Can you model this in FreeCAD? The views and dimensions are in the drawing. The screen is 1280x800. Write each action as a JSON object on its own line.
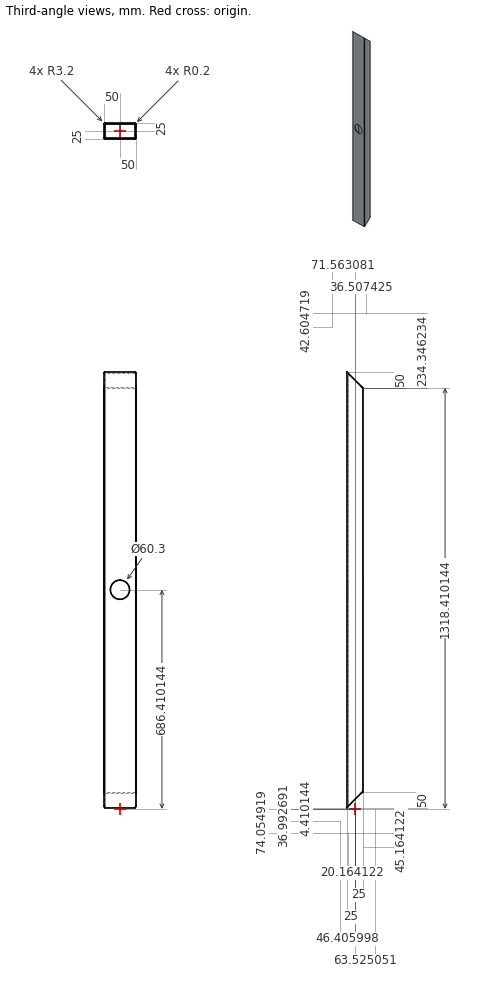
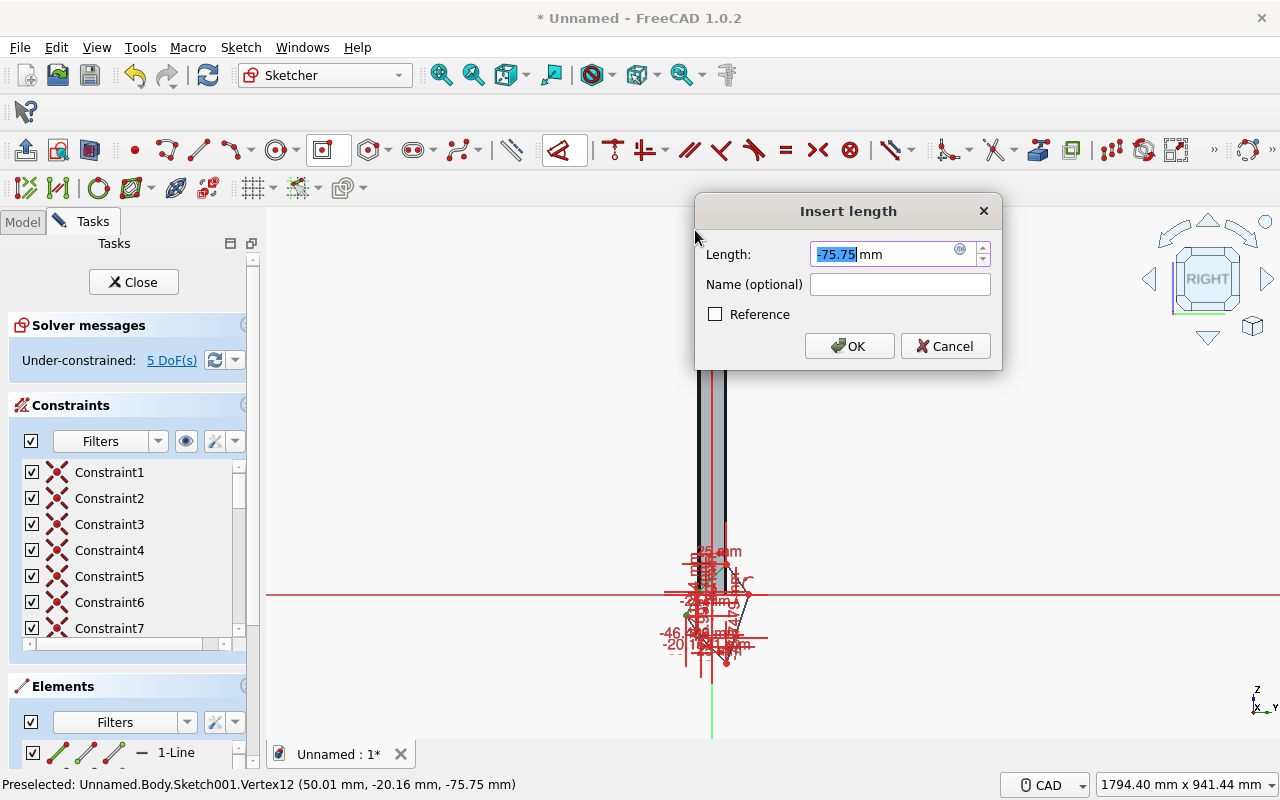
{"action": "type", "text": "-74.054919"}
{"action": "key", "text": "Return"}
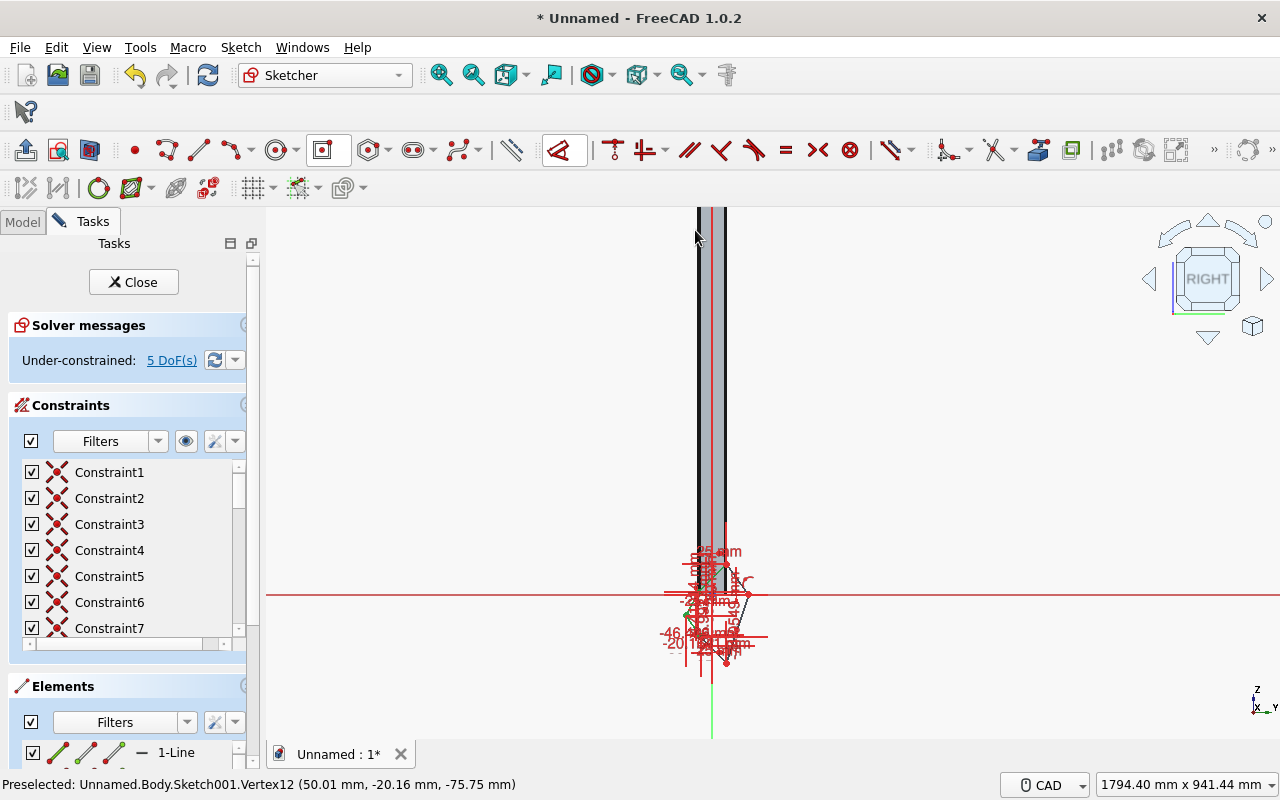
{"action": "left_click", "coordinate": [749, 595]}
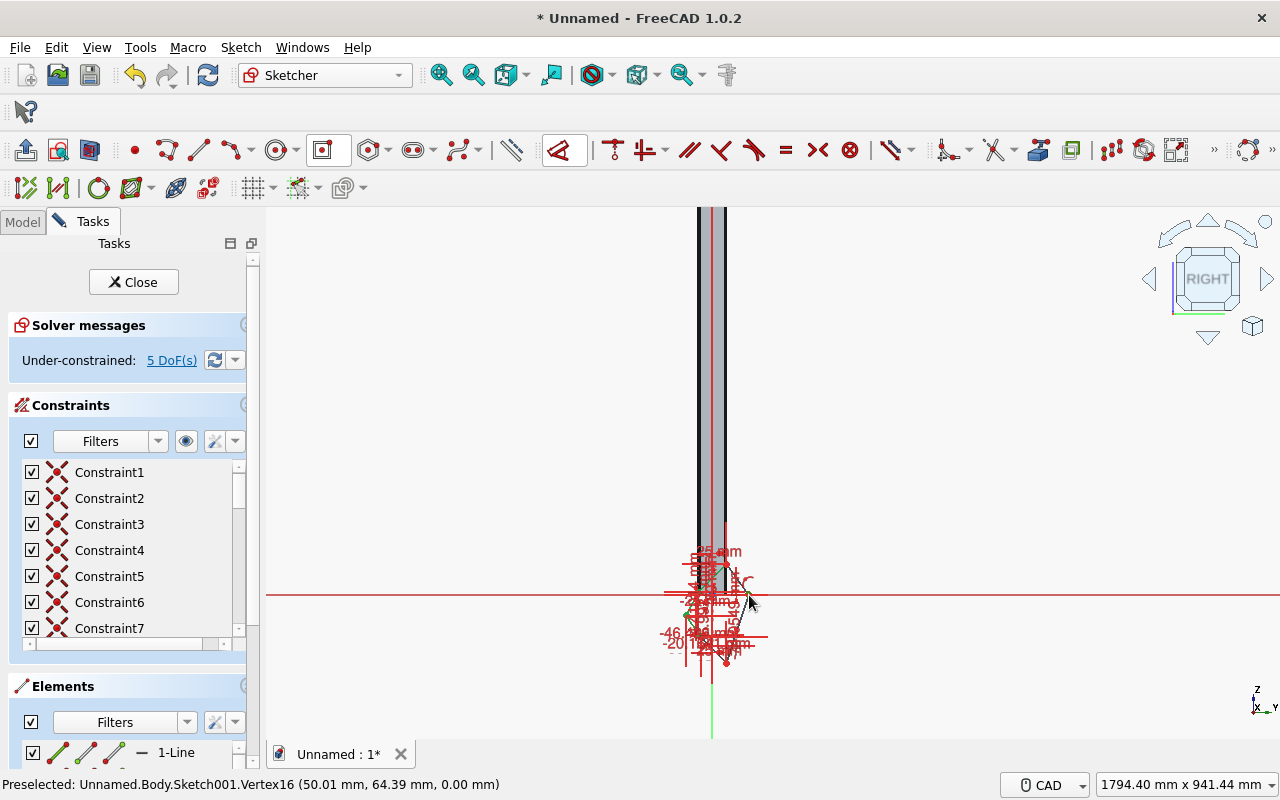
{"action": "left_click", "coordinate": [582, 150]}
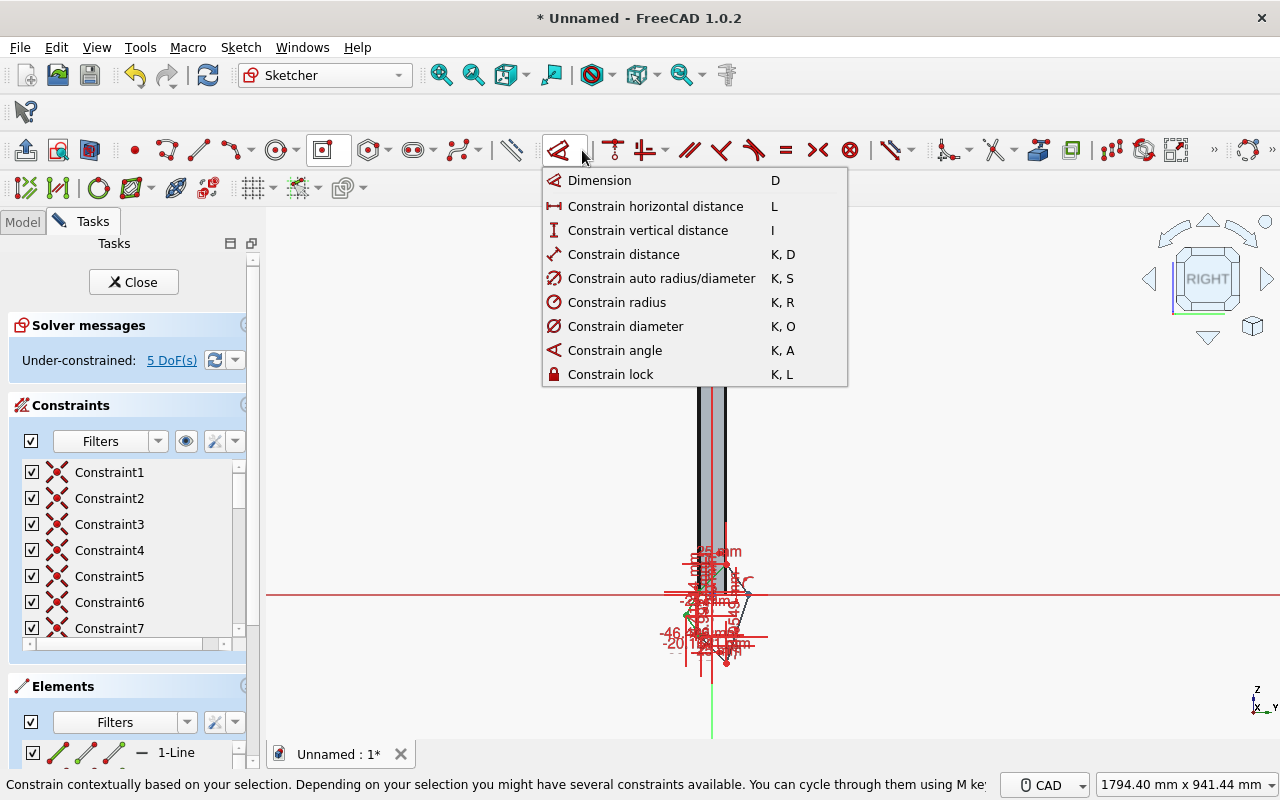
{"action": "left_click", "coordinate": [695, 206]}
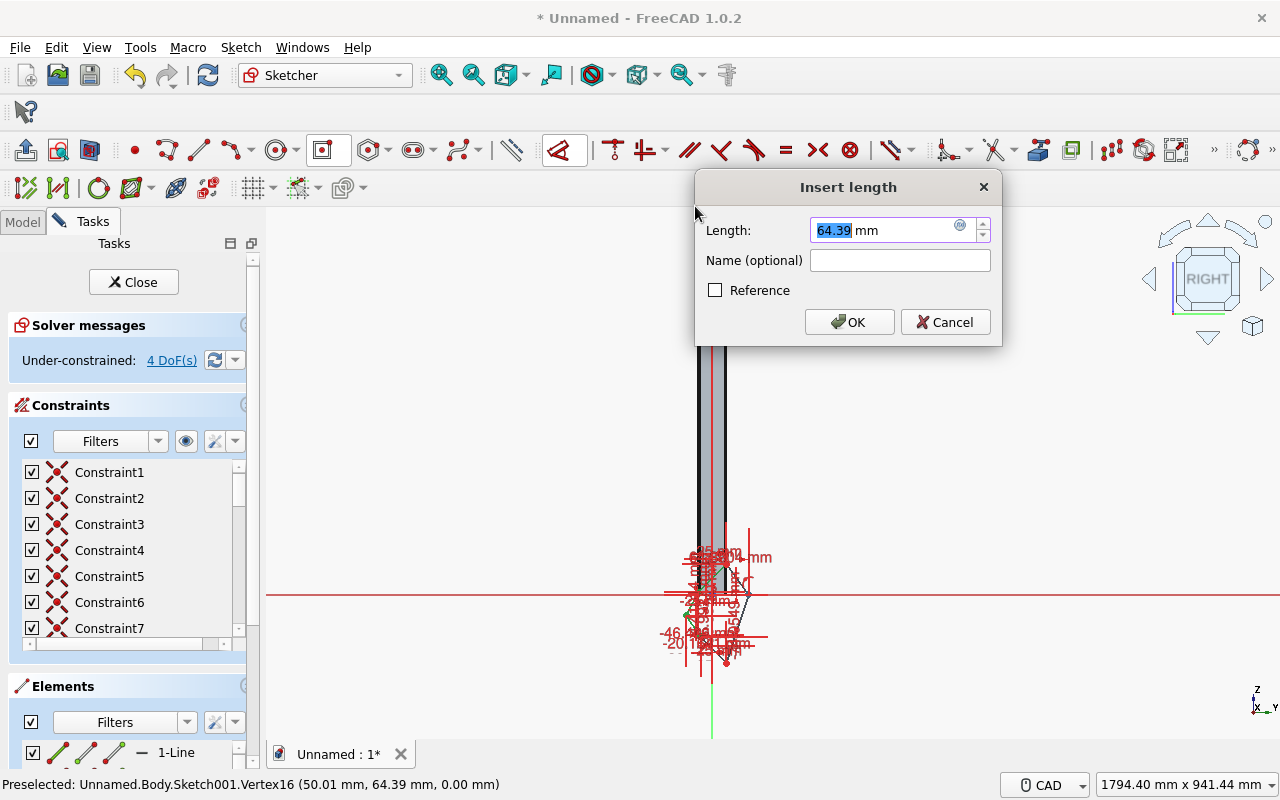
{"action": "type", "text": "63.525051"}
{"action": "key", "text": "Return"}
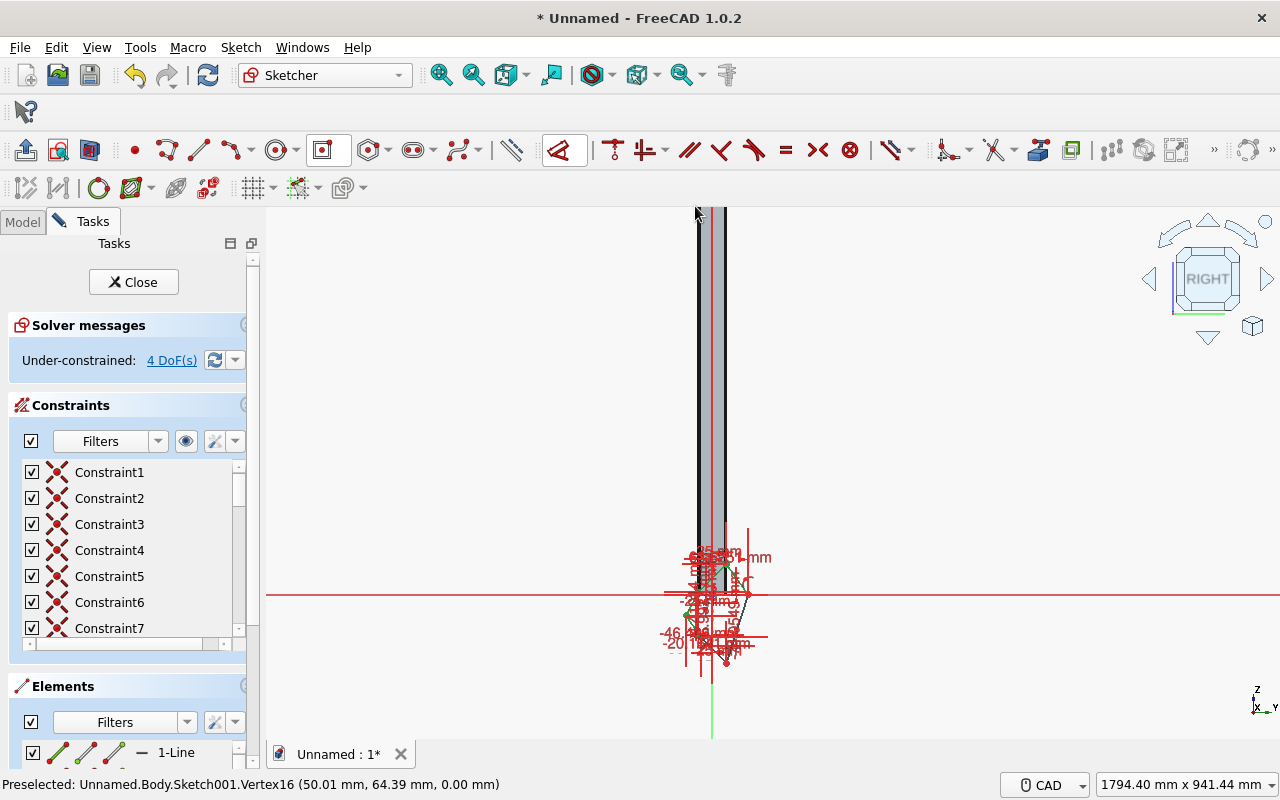
{"action": "scroll", "coordinate": [701, 638], "scroll_direction": "down", "scroll_amount": 5}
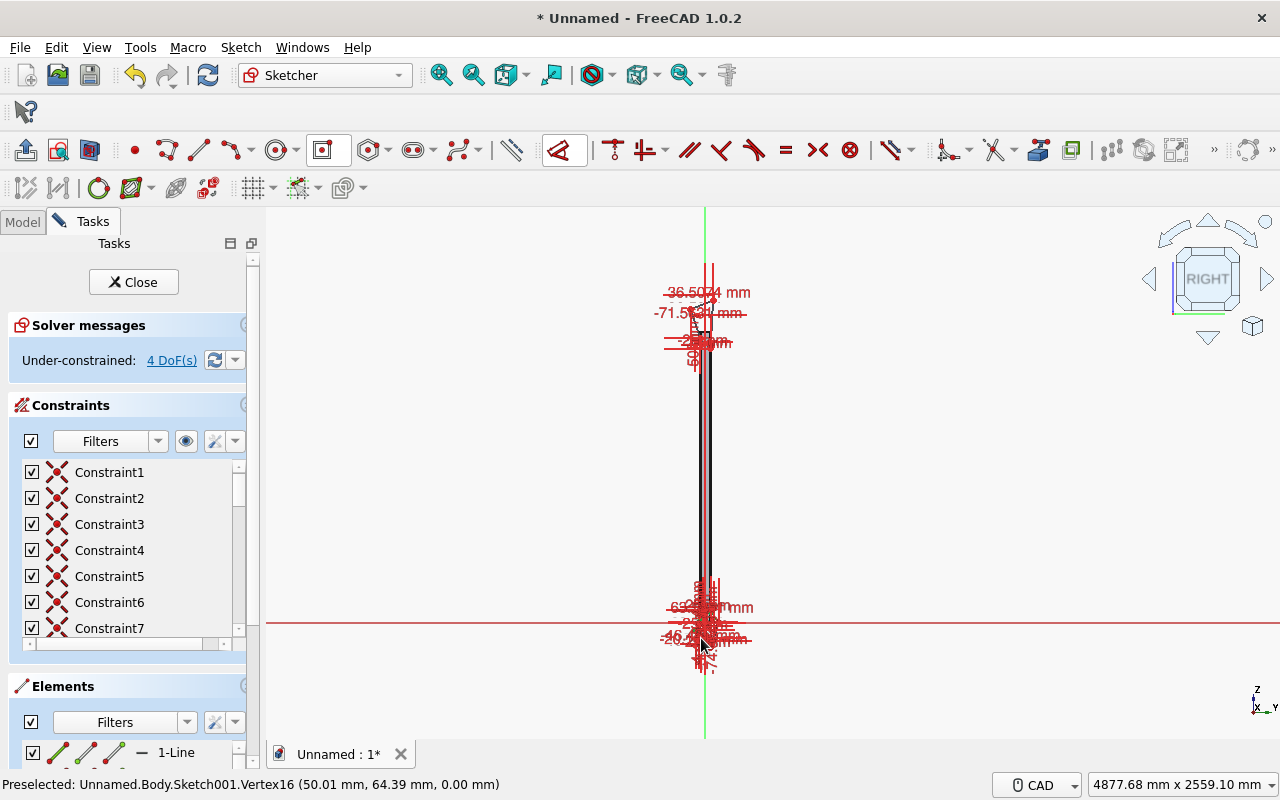
{"action": "scroll", "coordinate": [706, 303], "scroll_direction": "up", "scroll_amount": 8}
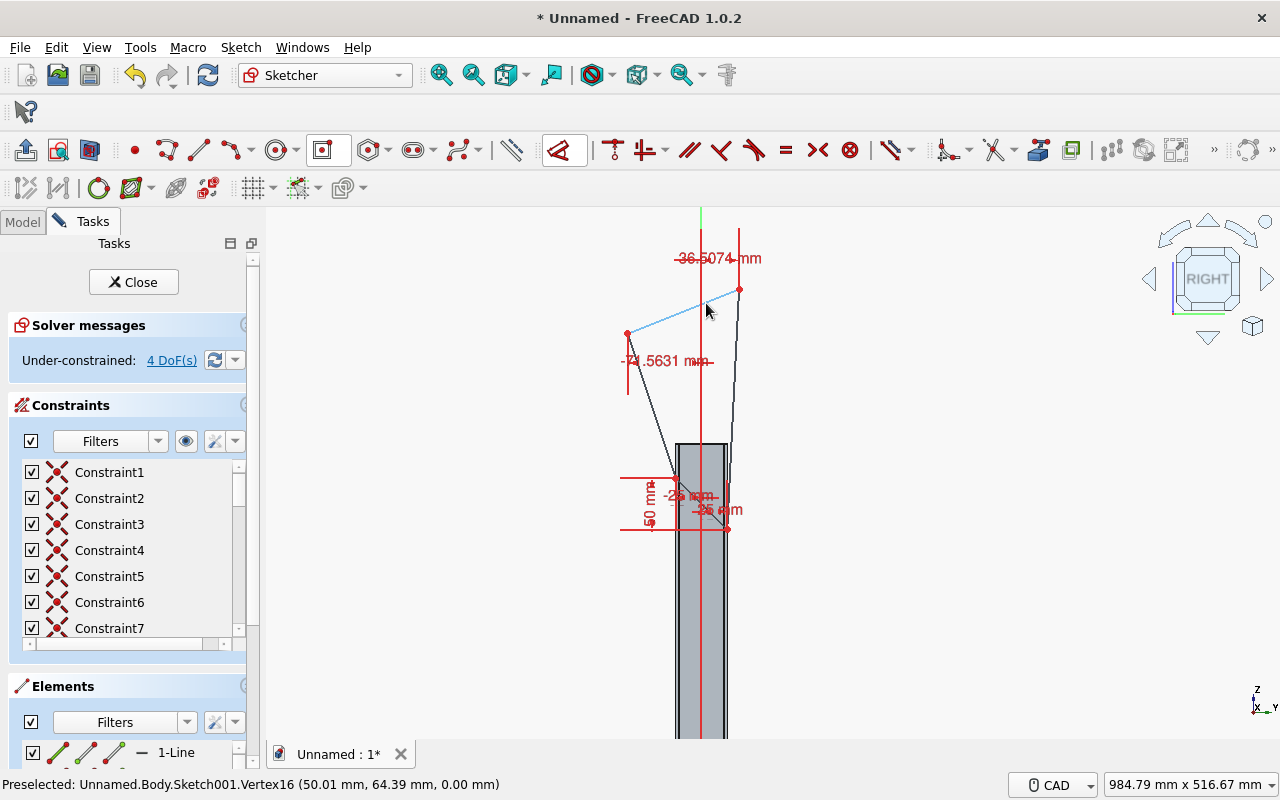
{"action": "left_click", "coordinate": [706, 303]}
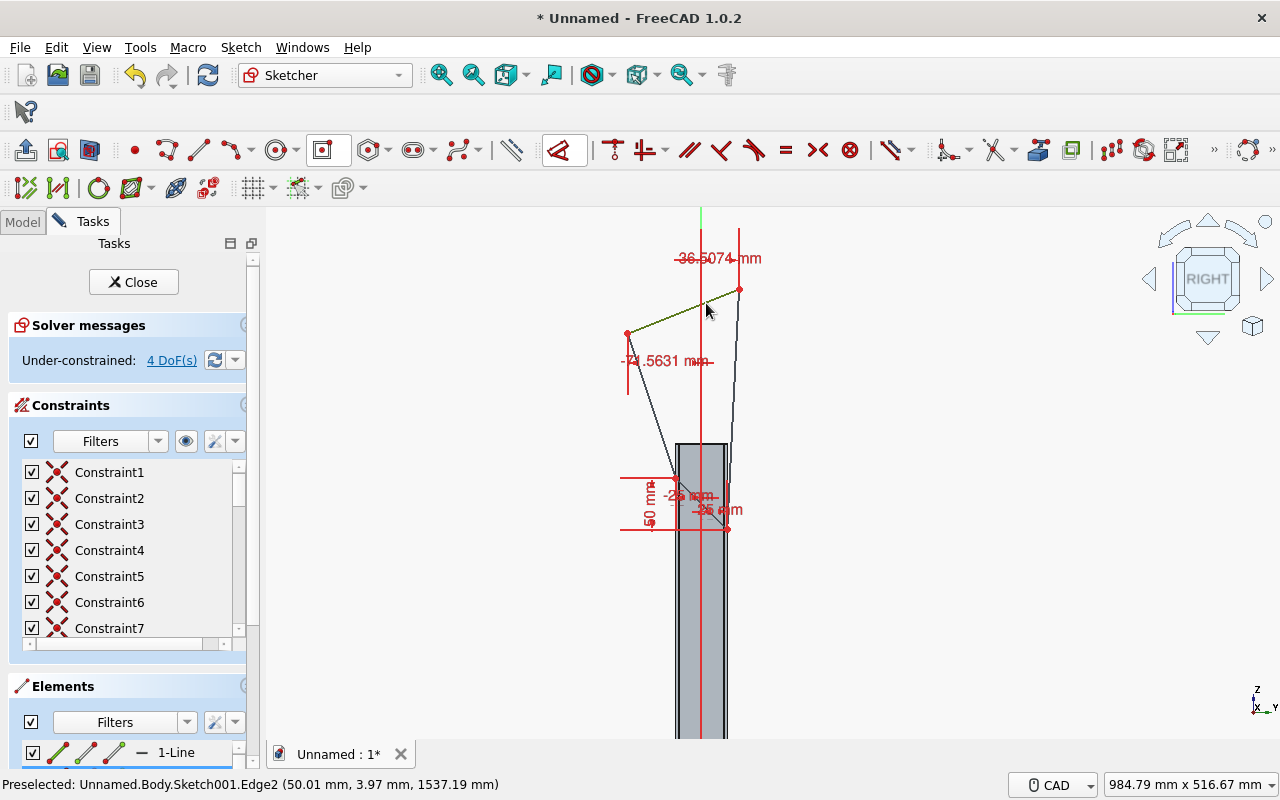
{"action": "left_click", "coordinate": [582, 150]}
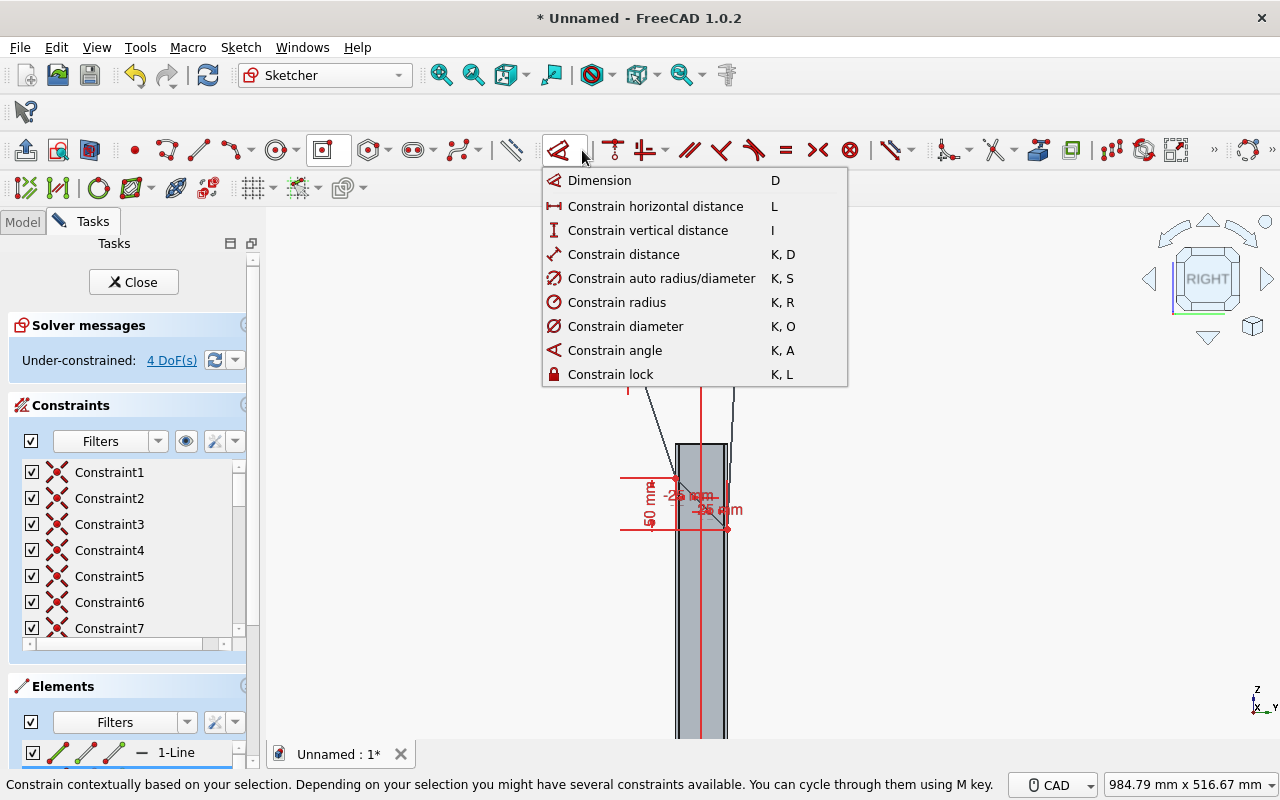
{"action": "left_click", "coordinate": [695, 230]}